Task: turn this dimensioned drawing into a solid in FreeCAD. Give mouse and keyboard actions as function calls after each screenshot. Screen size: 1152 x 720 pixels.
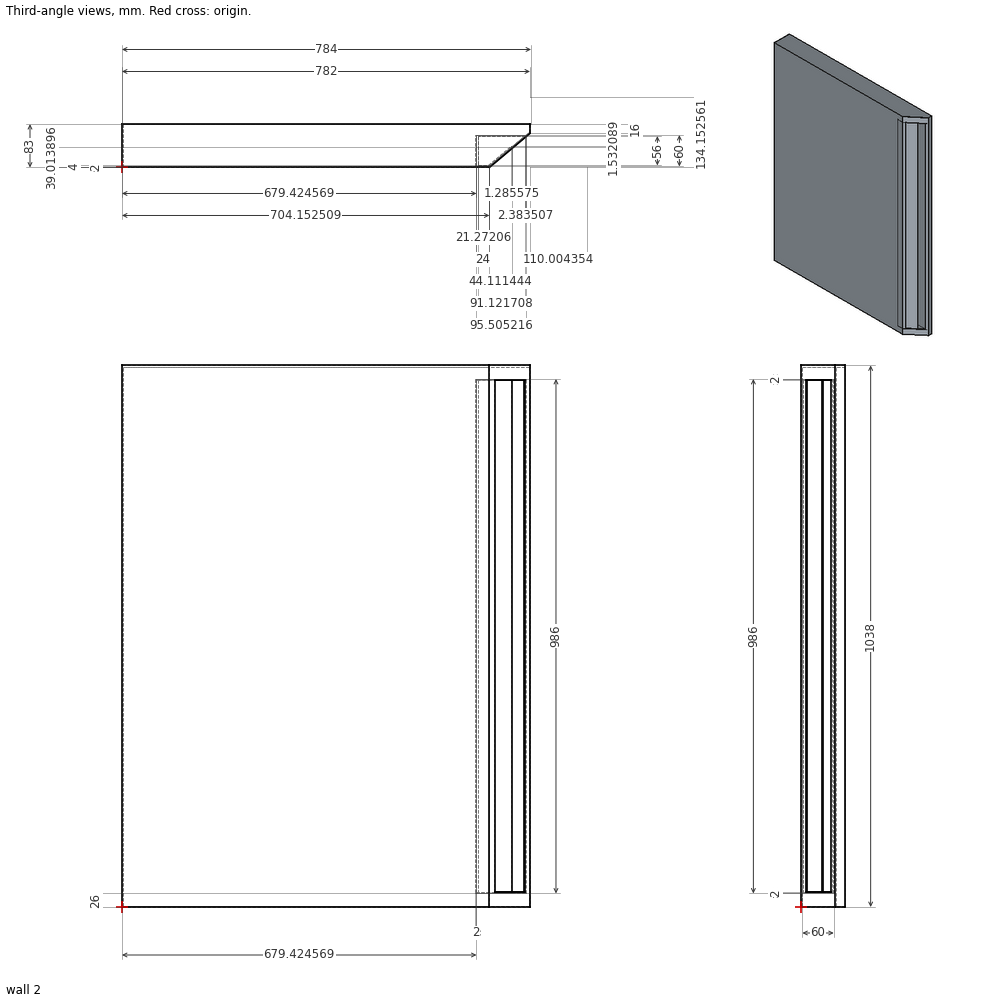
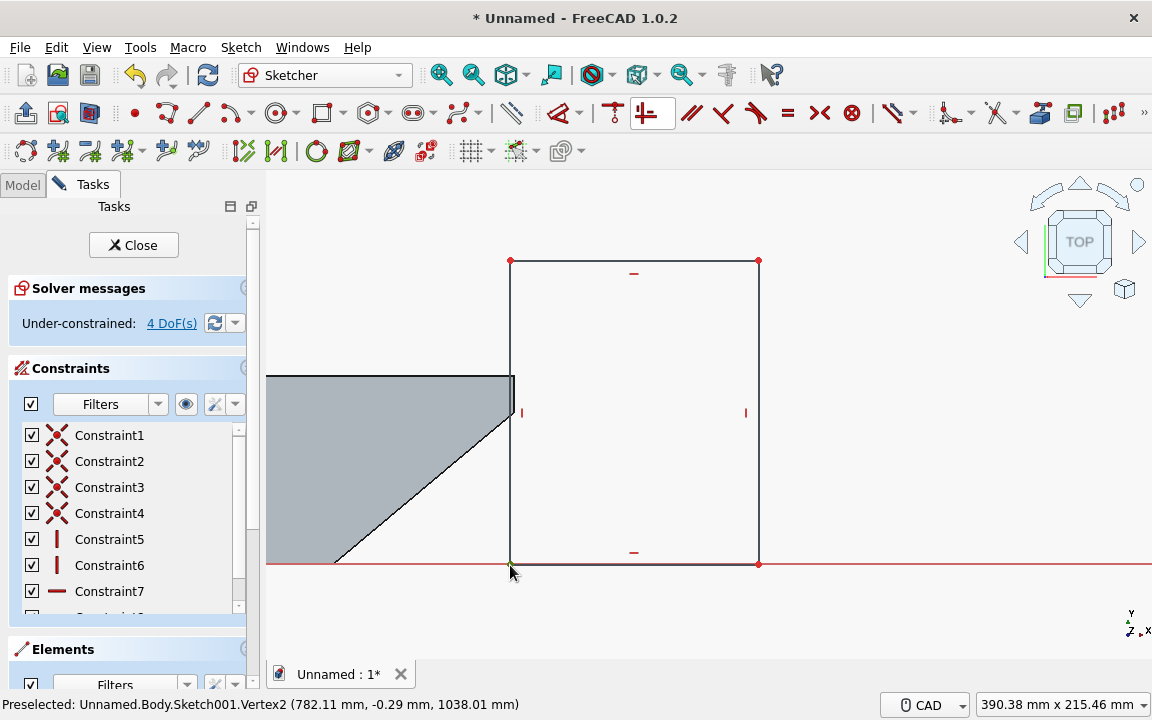
click(343, 564)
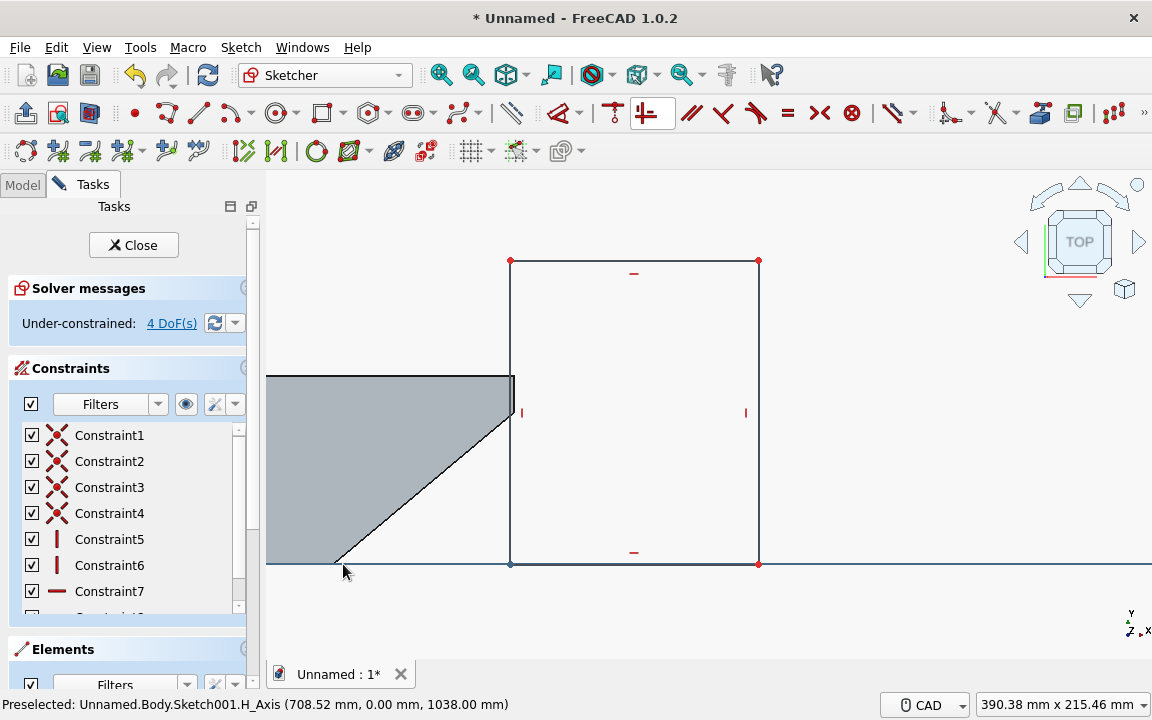
click(614, 114)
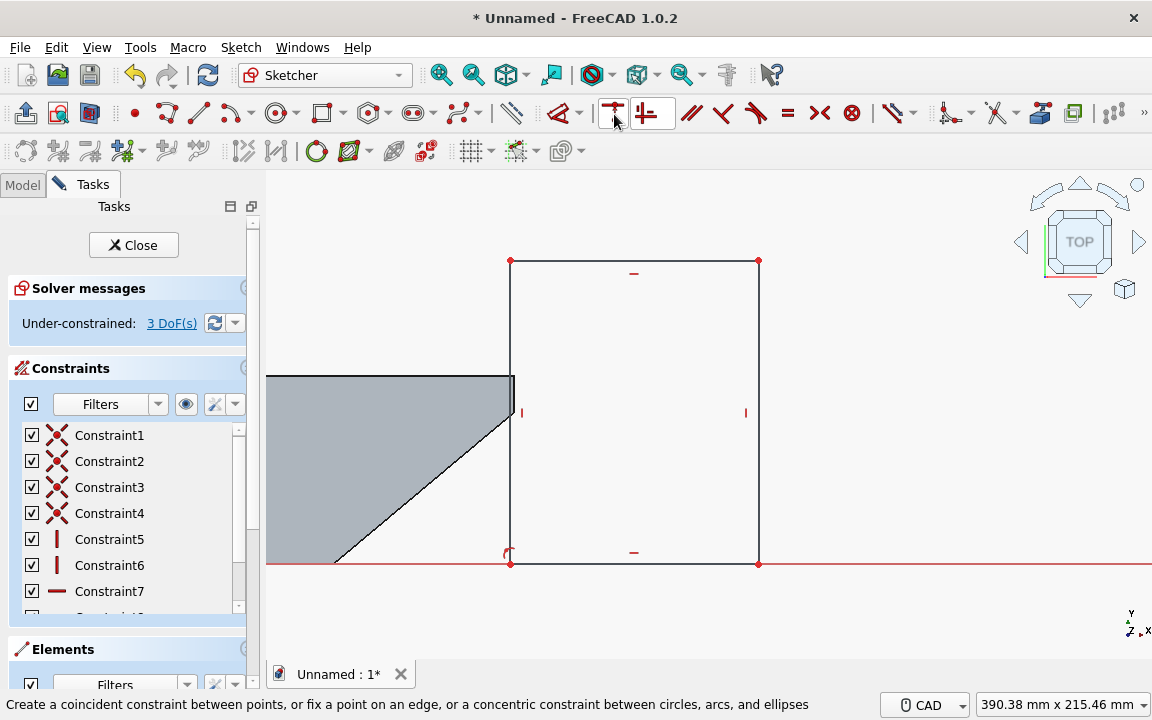
click(558, 114)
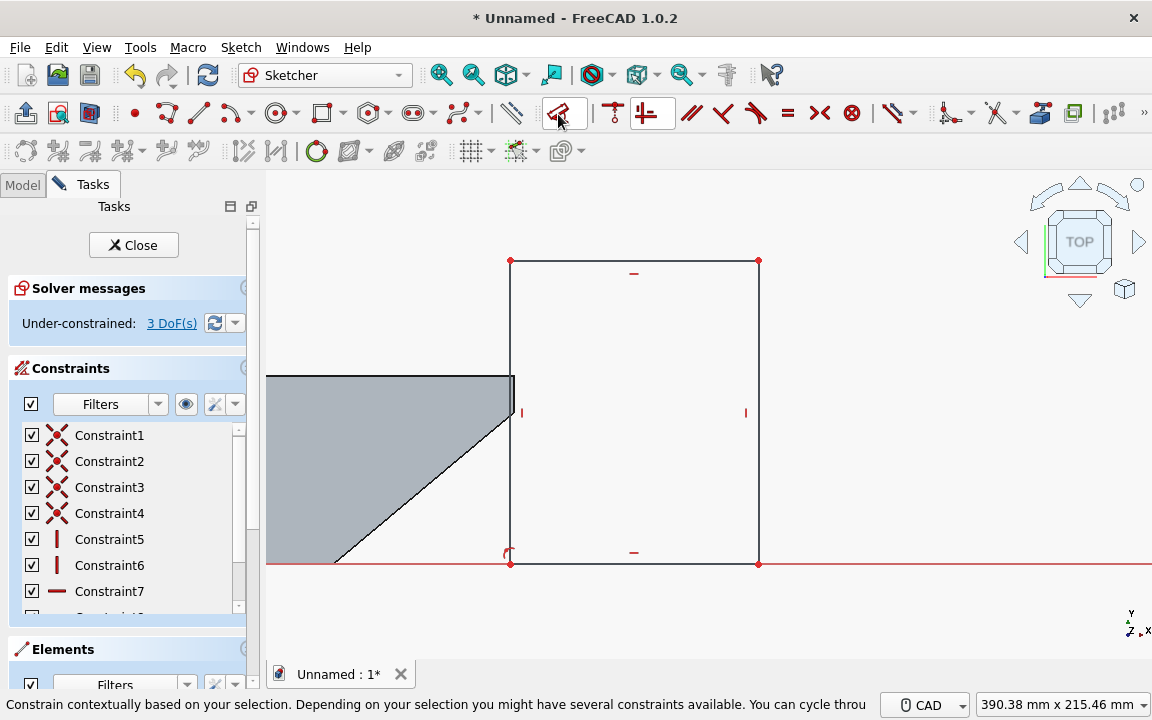
click(510, 261)
click(402, 598)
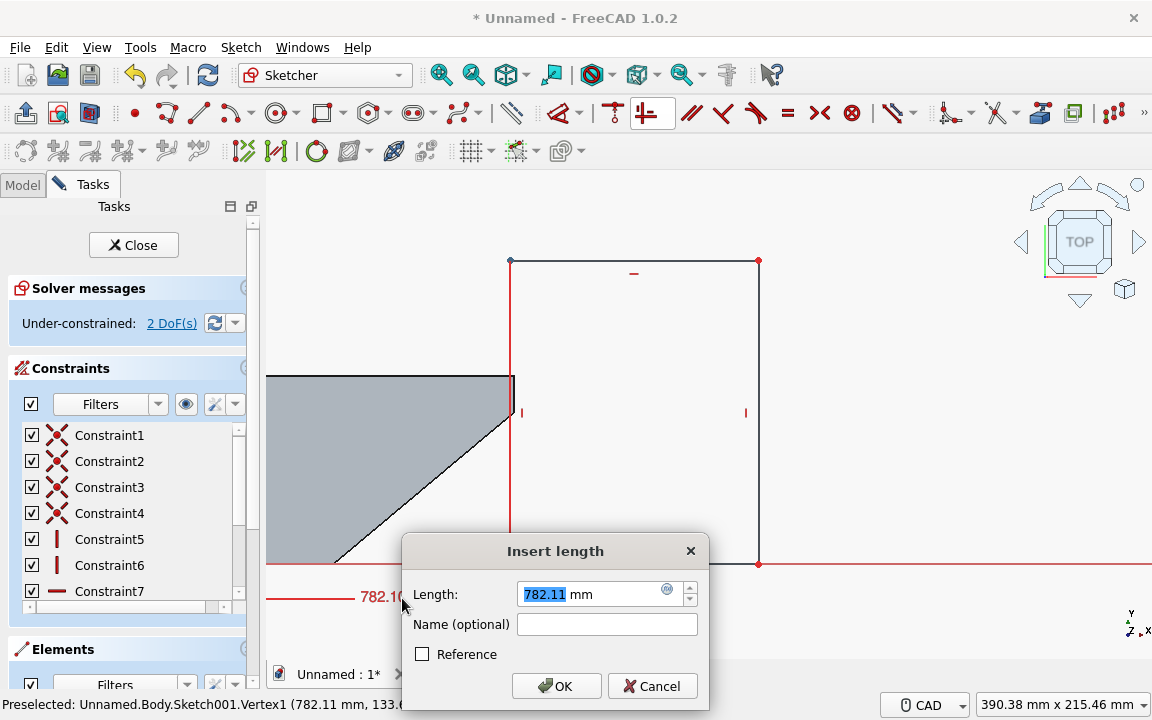
text(782)
key(Return)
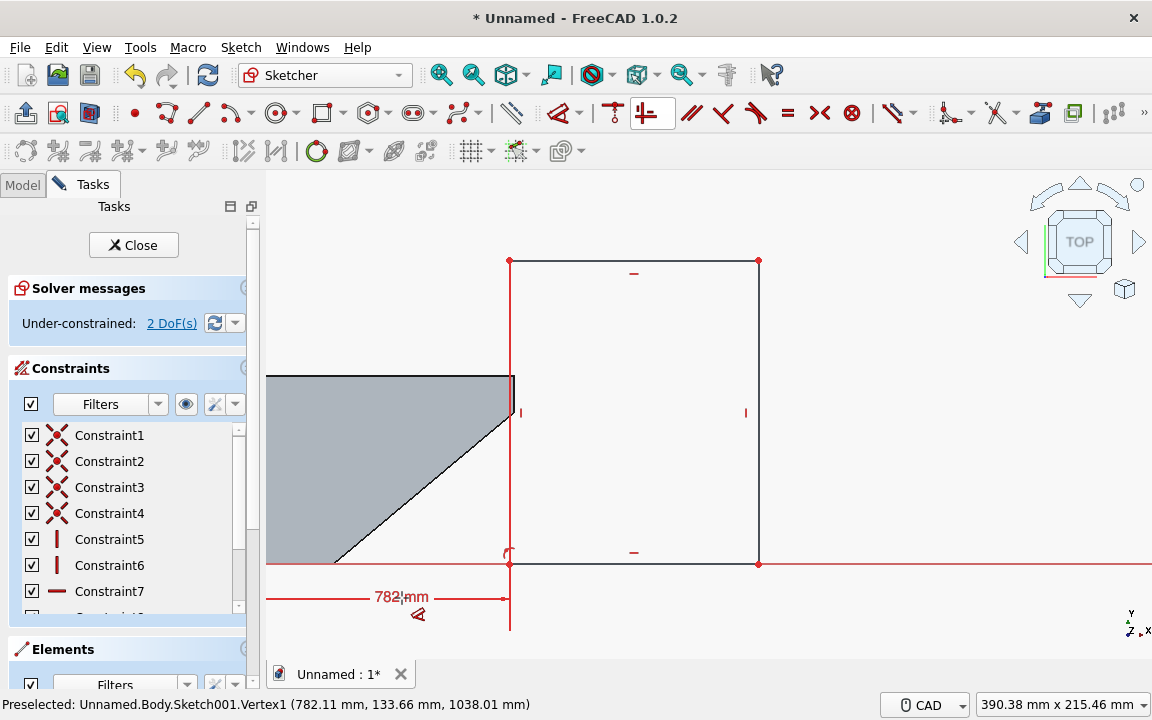
click(510, 352)
click(476, 413)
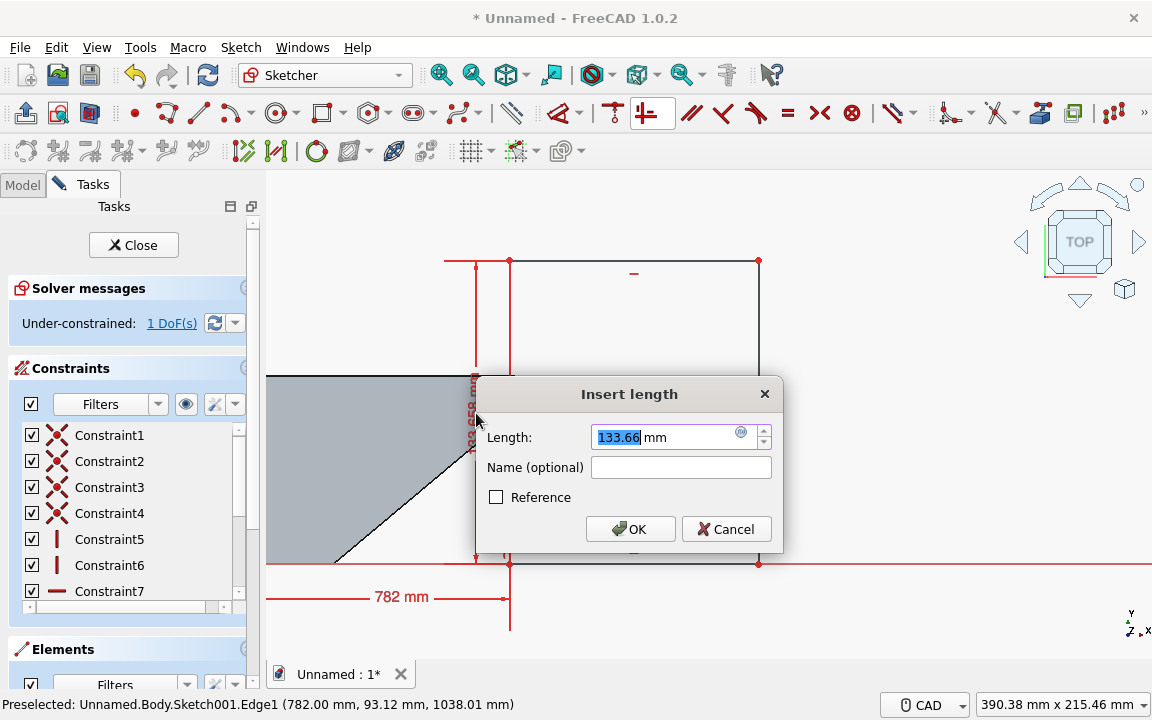
text(134.152561)
key(Return)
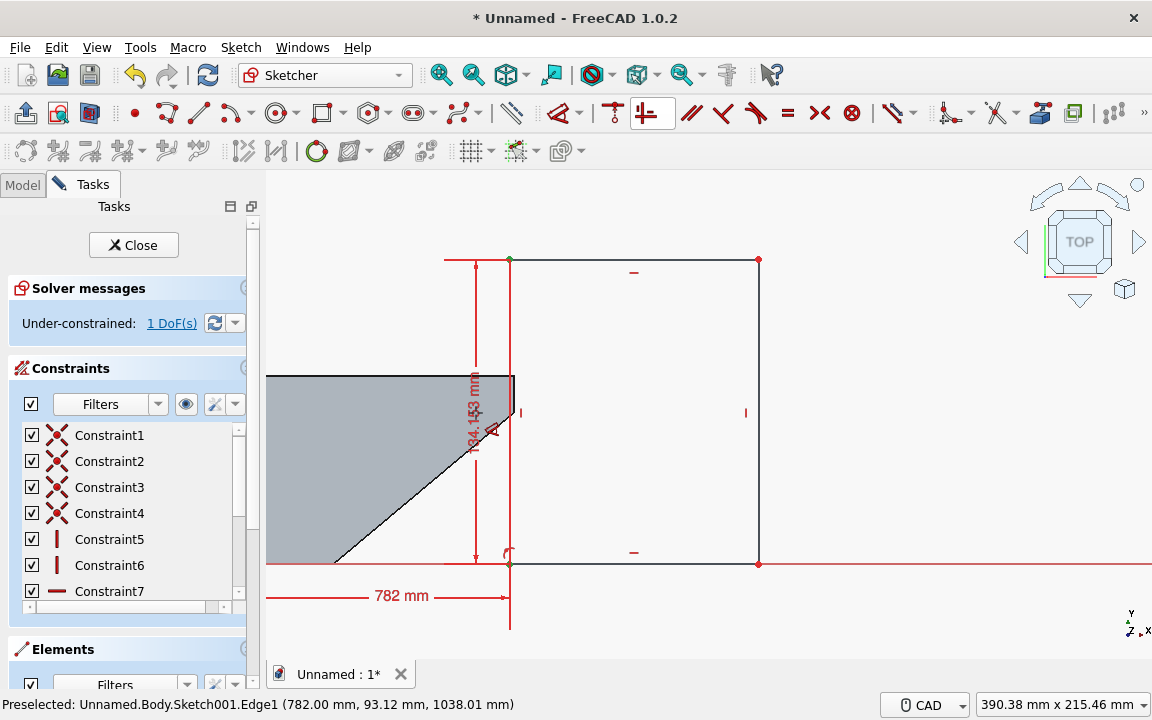
click(585, 564)
click(634, 598)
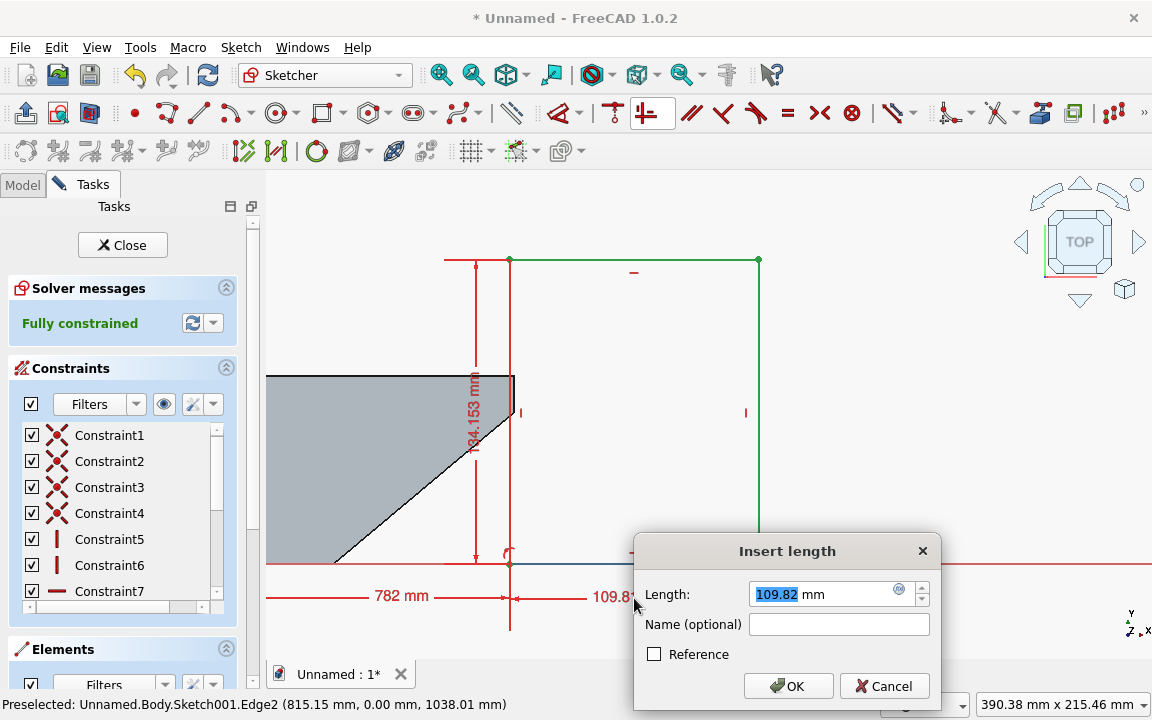
text(110.004354)
key(Return)
key(Escape)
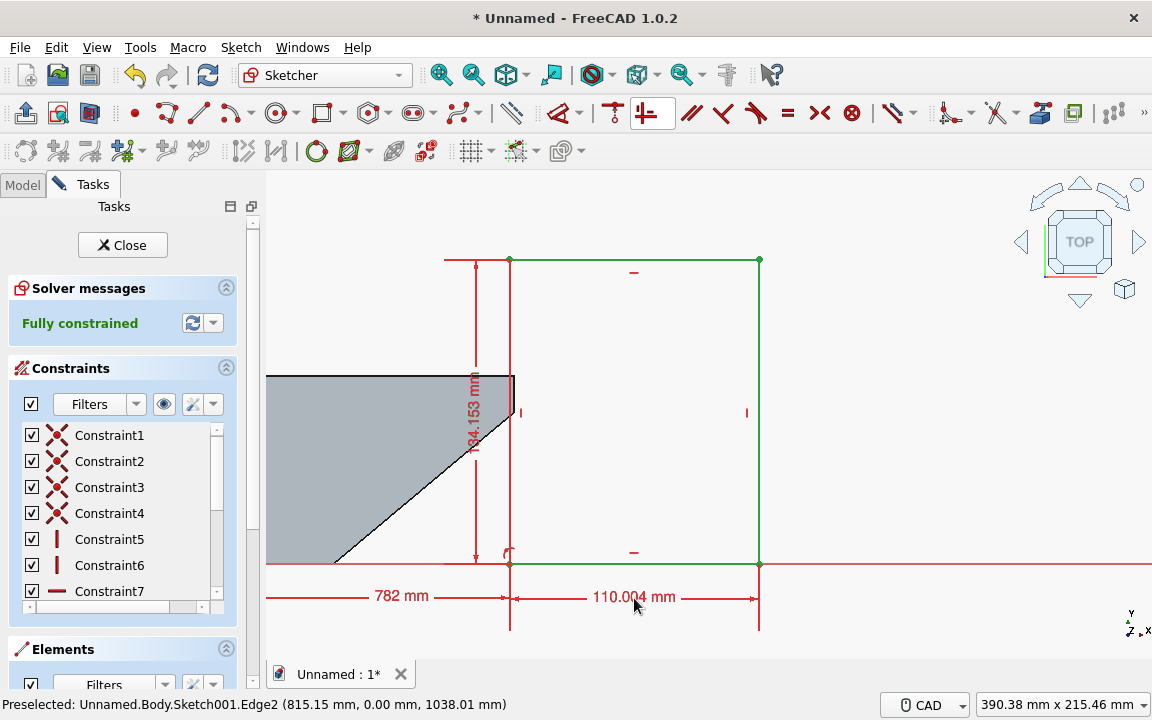
click(123, 245)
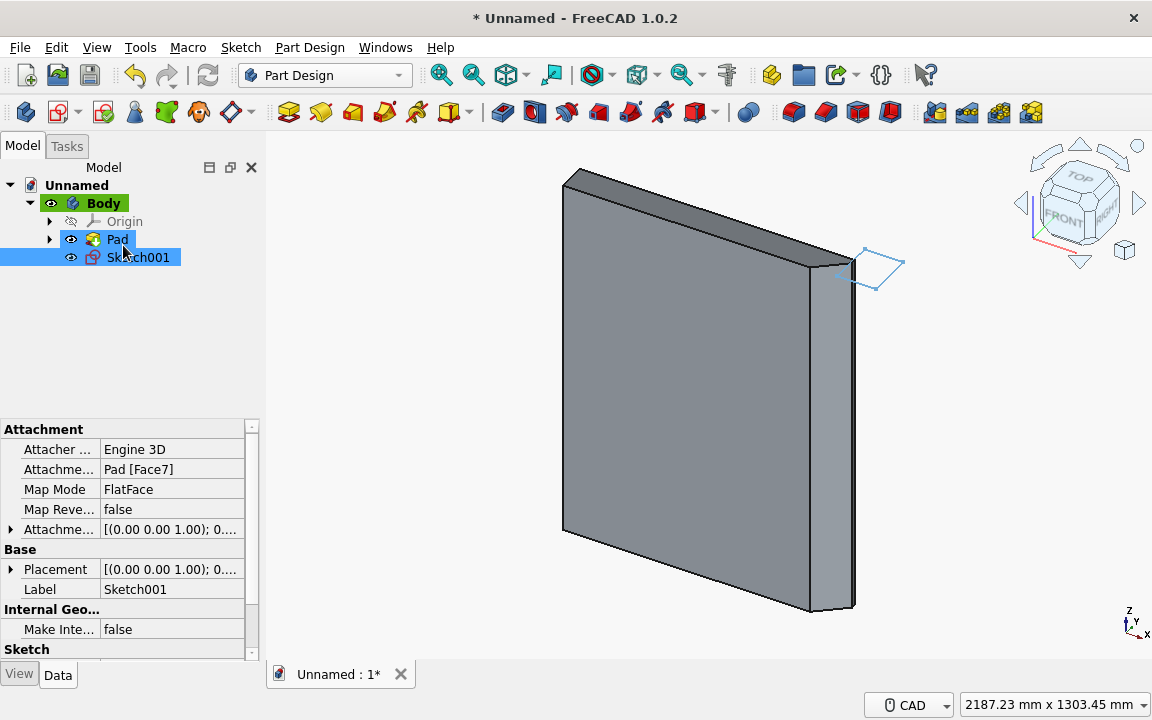
click(504, 112)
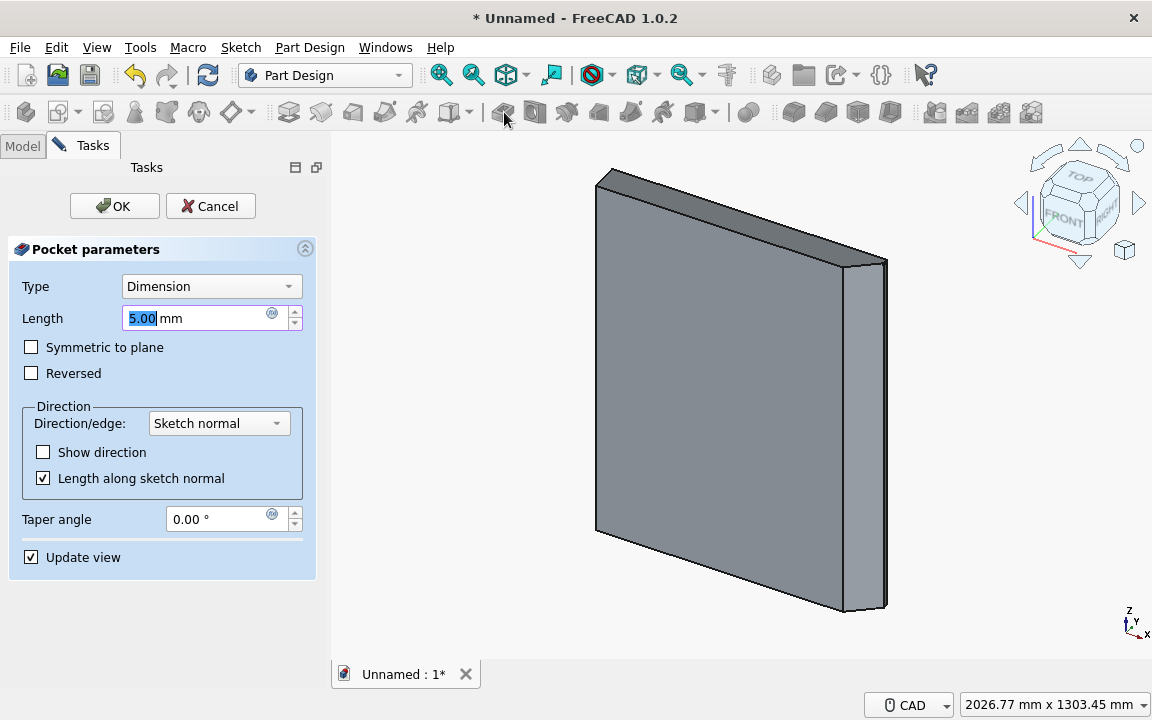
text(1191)
key(Tab)